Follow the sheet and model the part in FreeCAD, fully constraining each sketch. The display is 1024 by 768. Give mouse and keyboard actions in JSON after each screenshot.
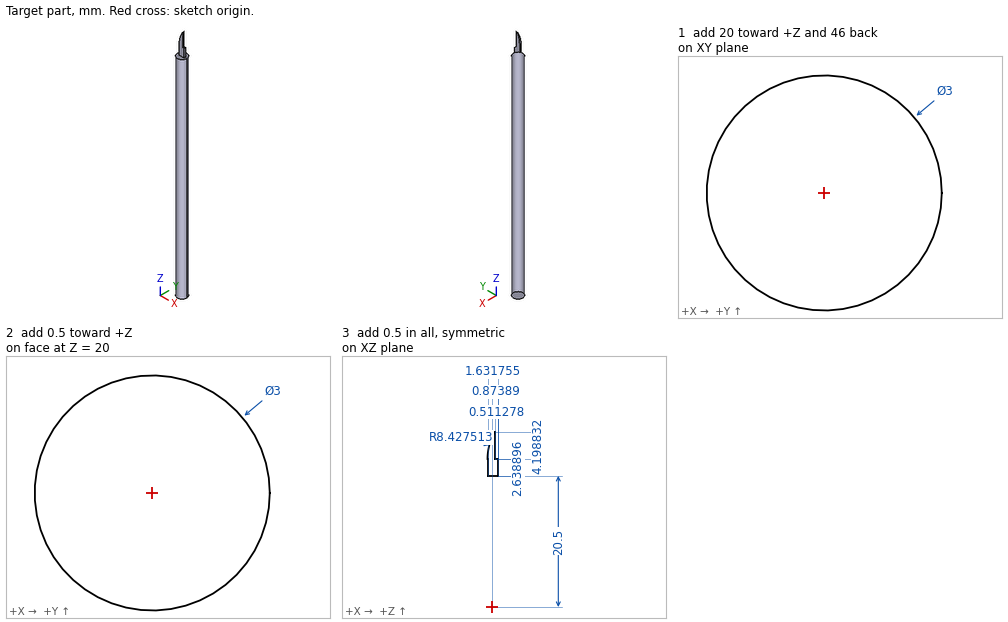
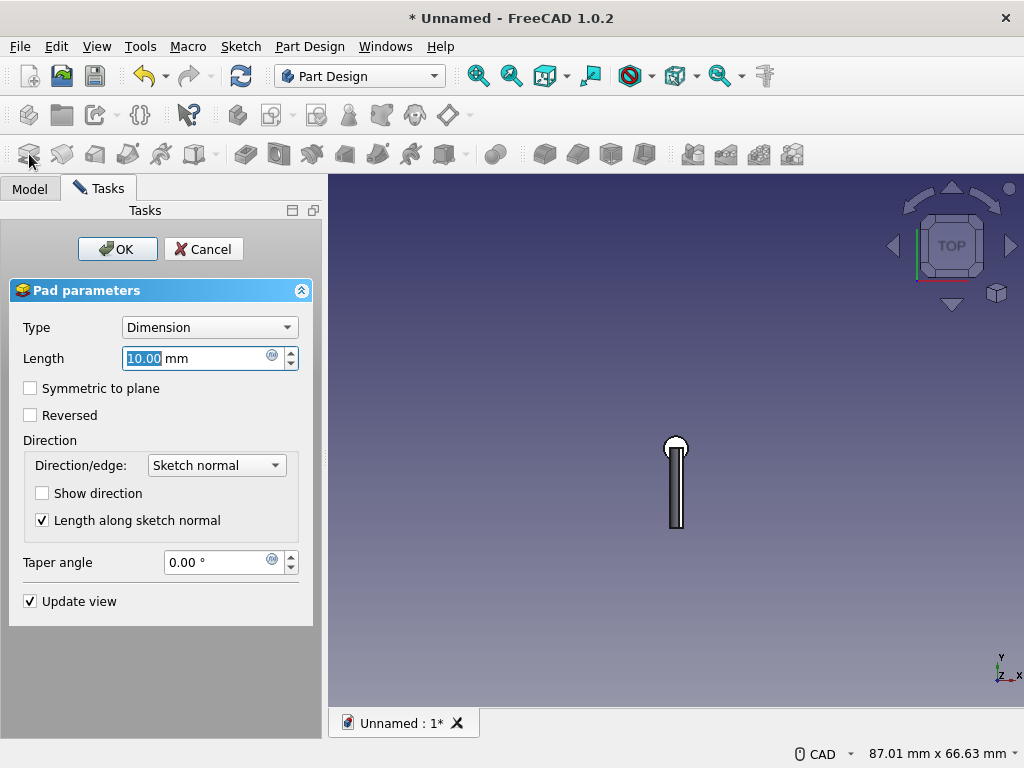
{"action": "type", "text": "0.5"}
{"action": "key", "text": "Tab"}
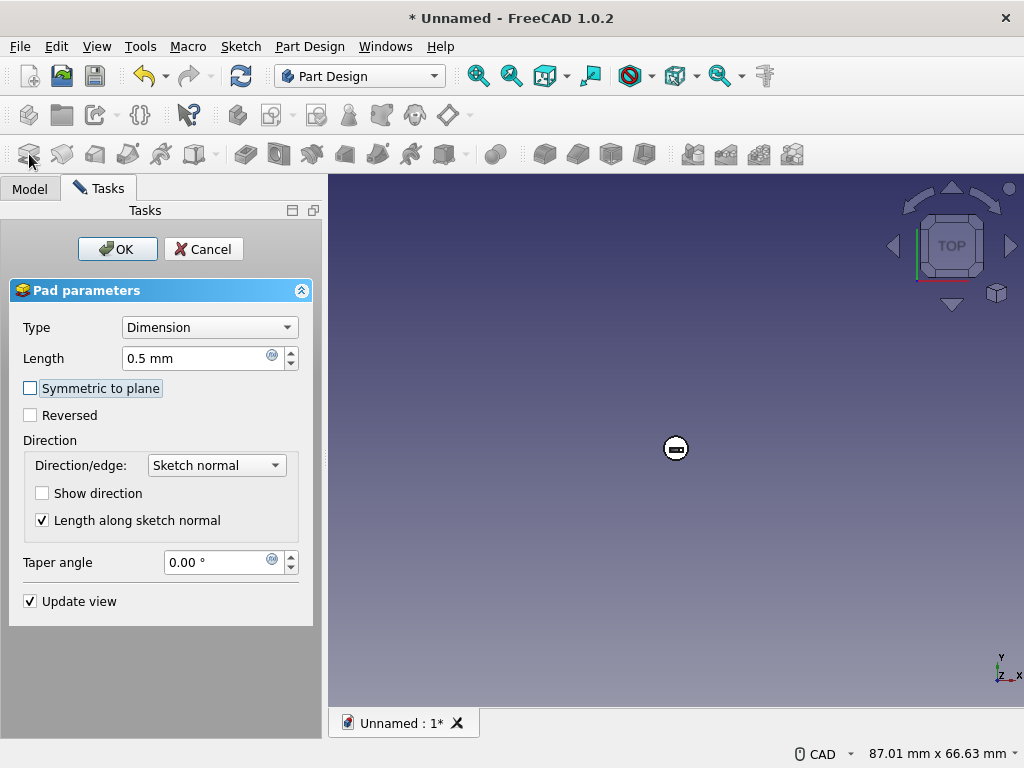
{"action": "left_click", "coordinate": [31, 388]}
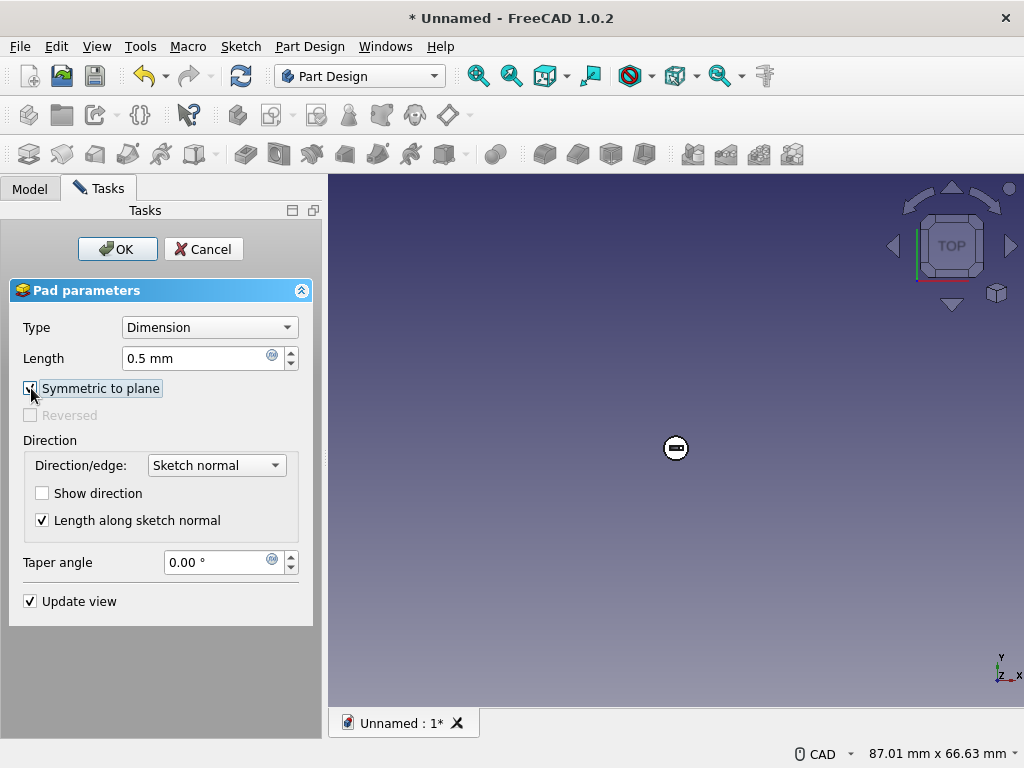
{"action": "left_click", "coordinate": [118, 249]}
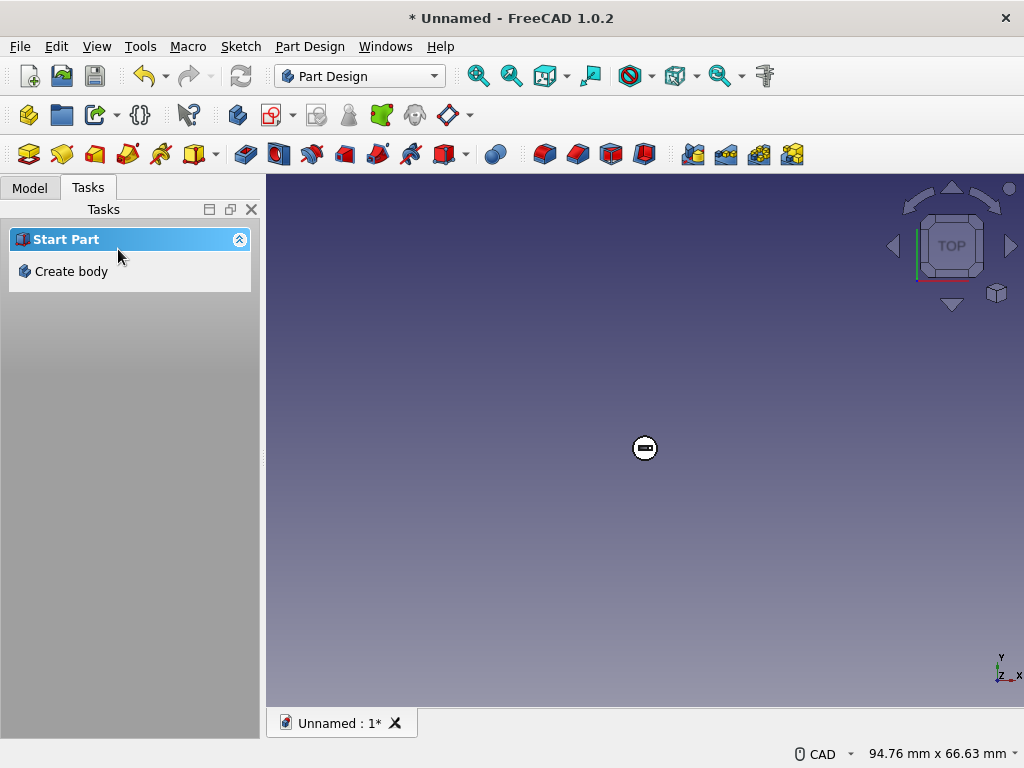
{"action": "key", "text": "0"}